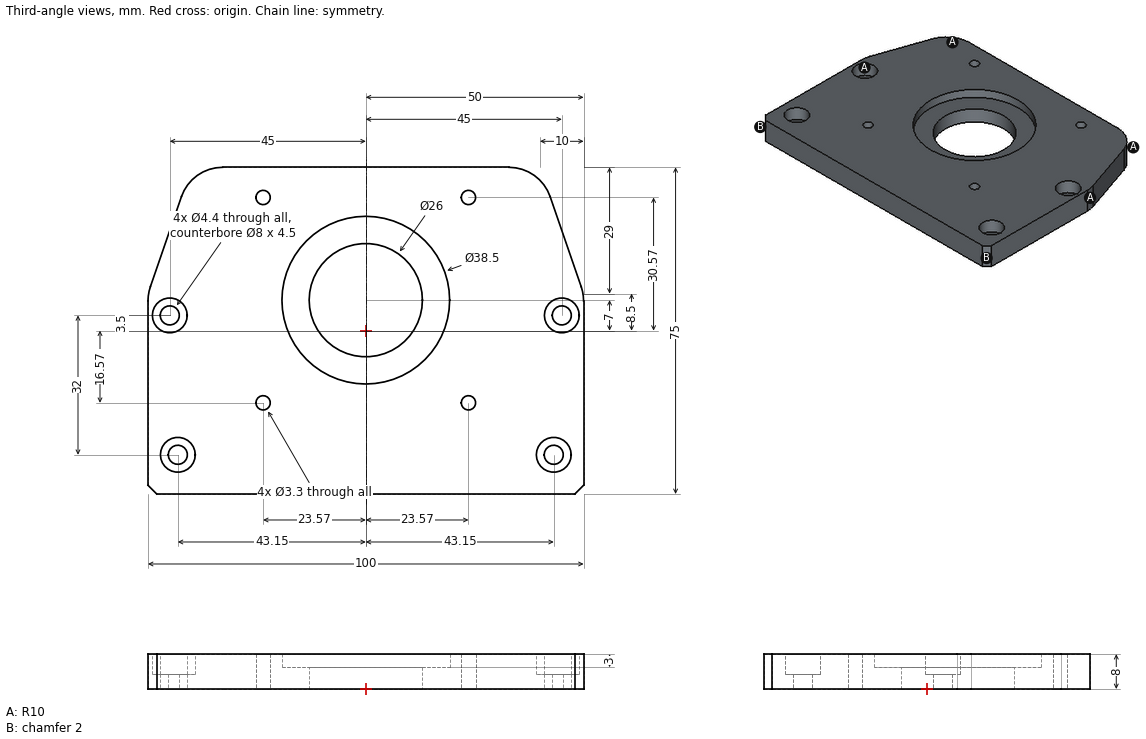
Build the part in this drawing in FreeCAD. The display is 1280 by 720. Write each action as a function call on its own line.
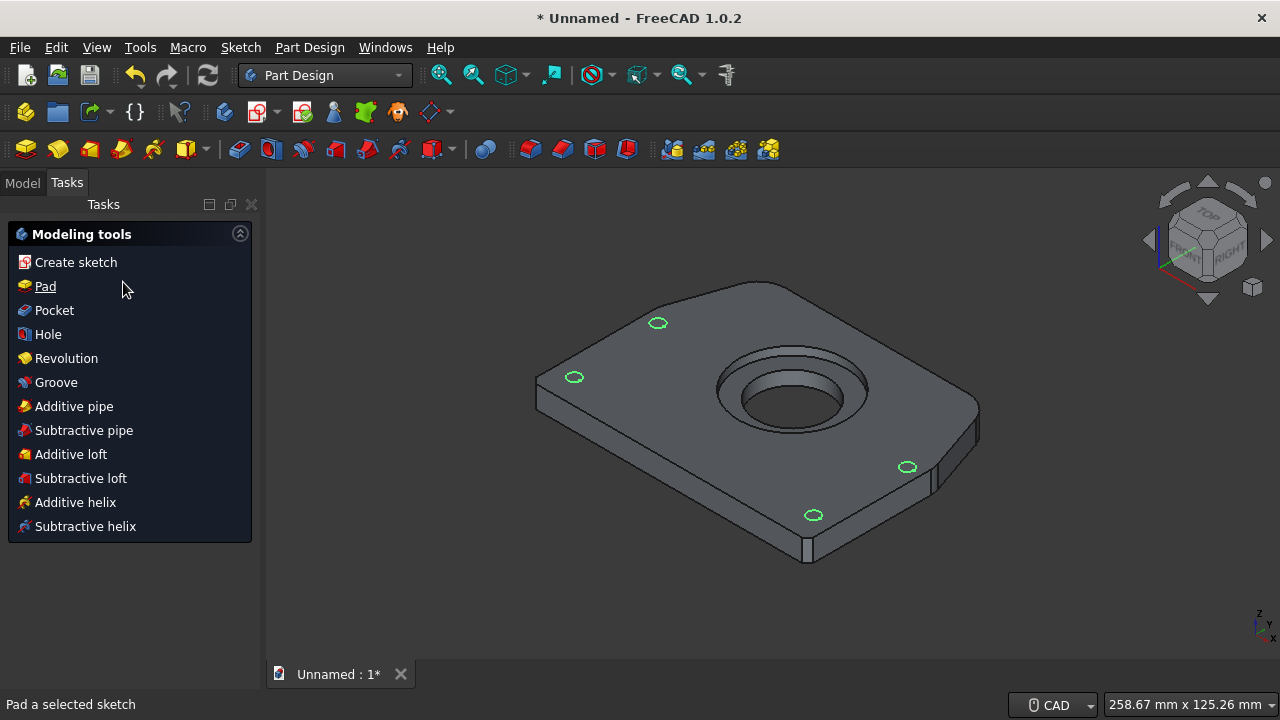
click(272, 150)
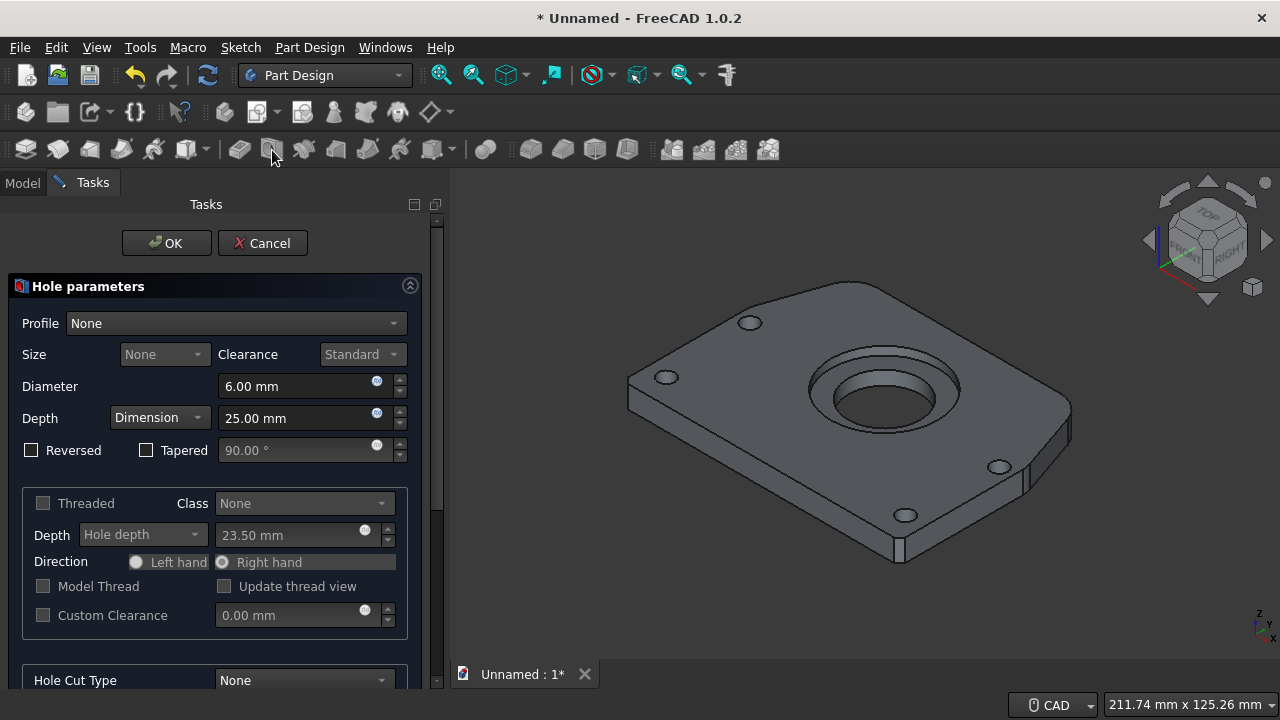
triple_click(305, 386)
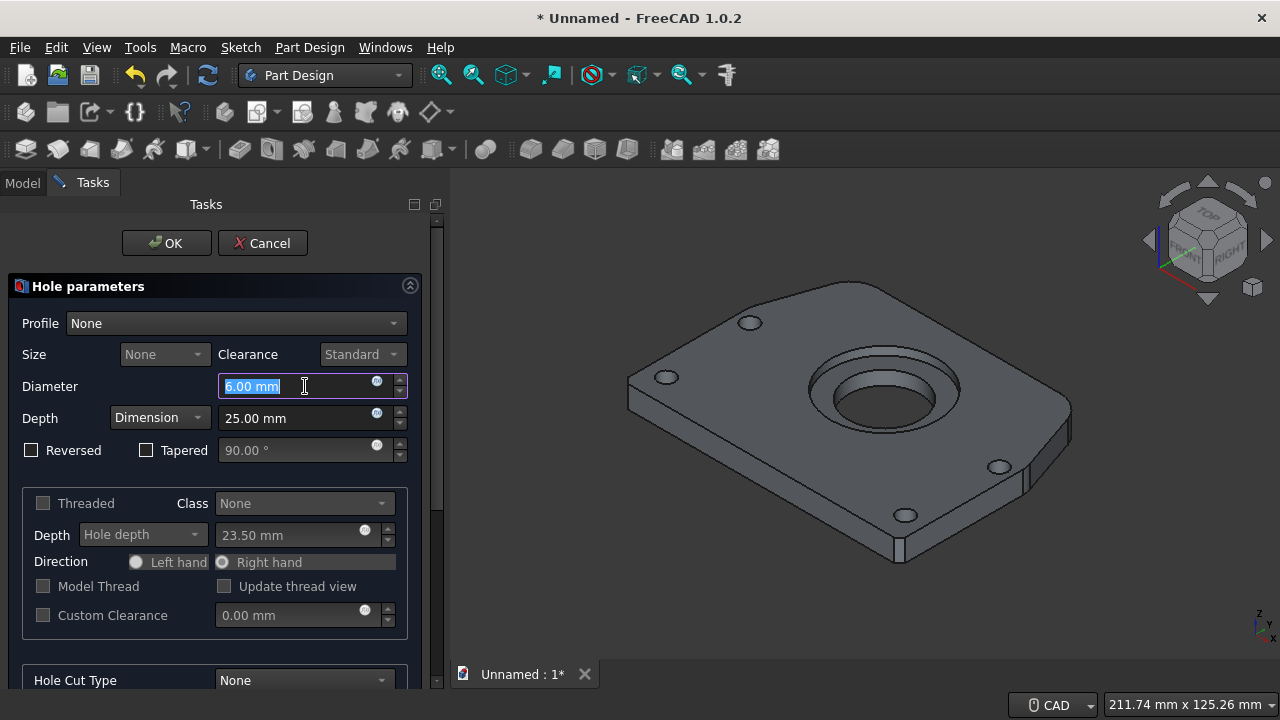
text(4.4)
key(Tab)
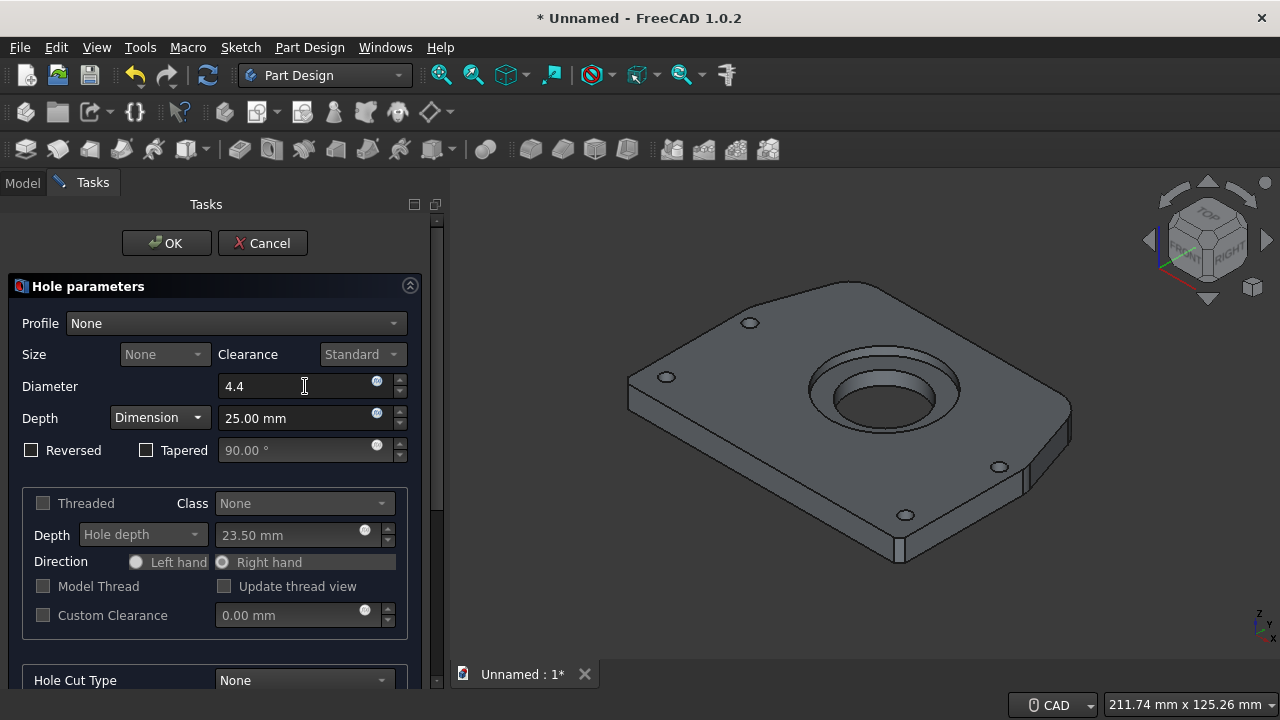
click(161, 418)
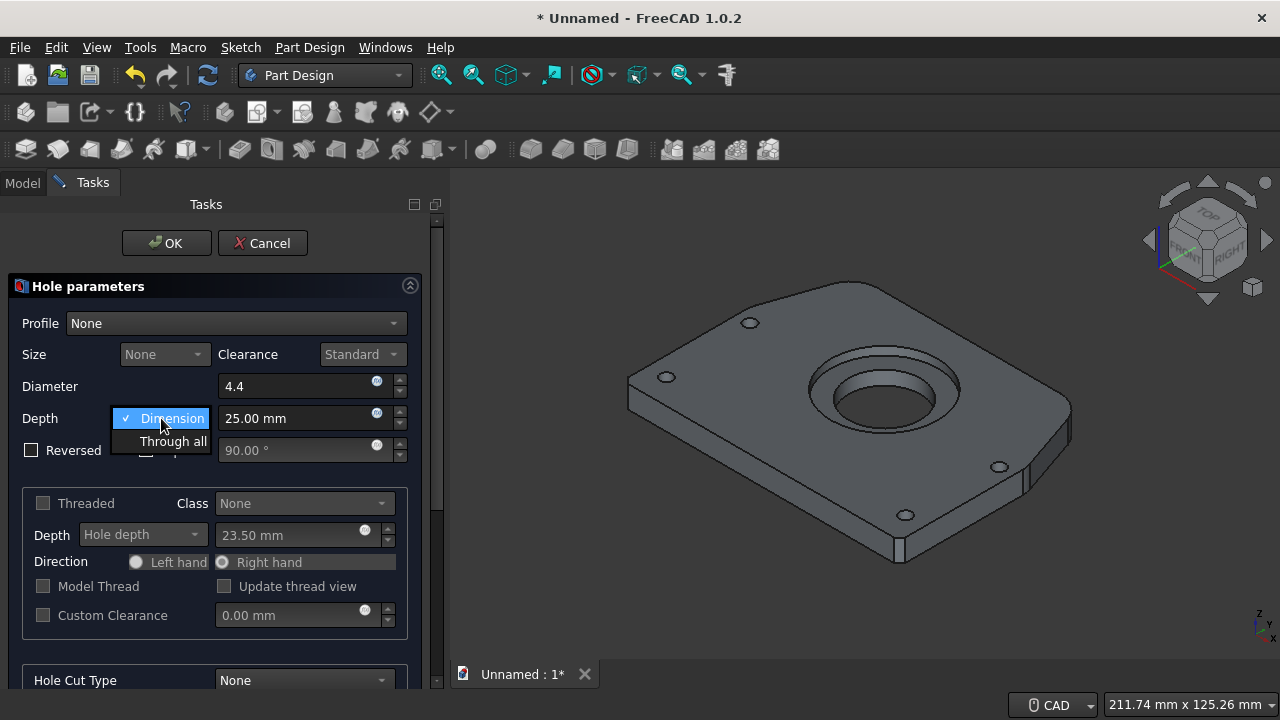
click(160, 442)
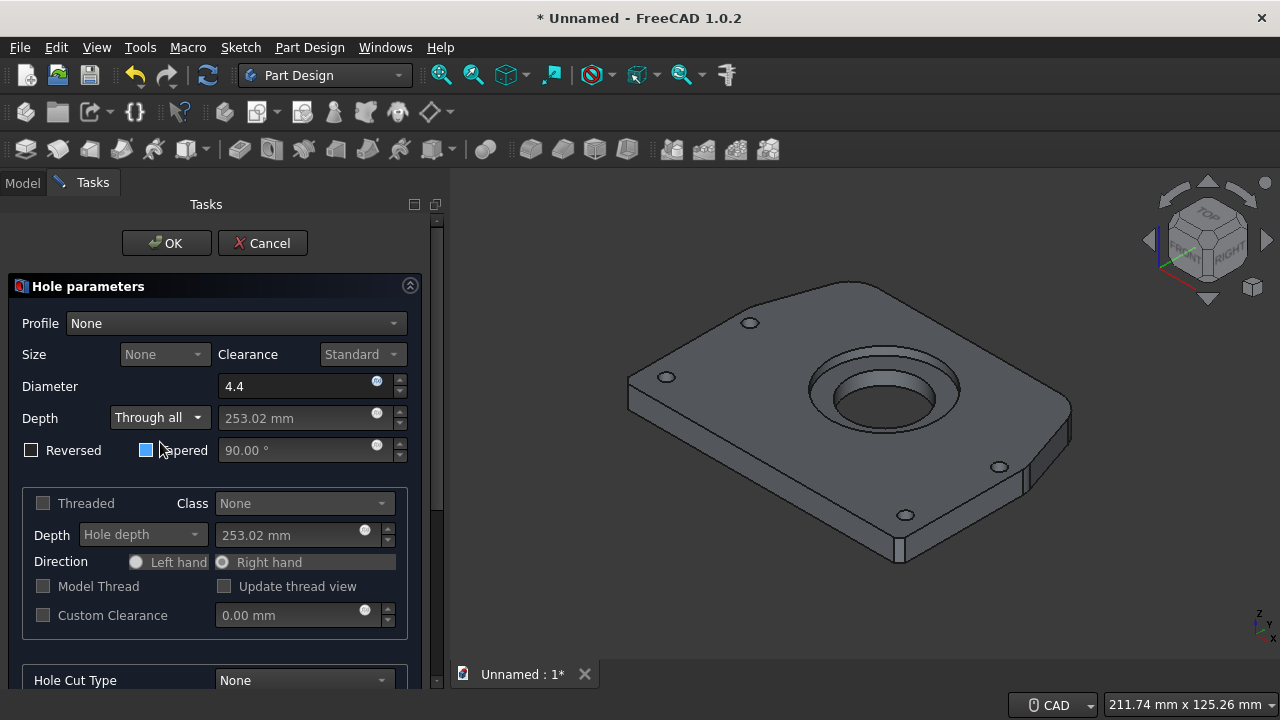
scroll(437, 451, down, 2)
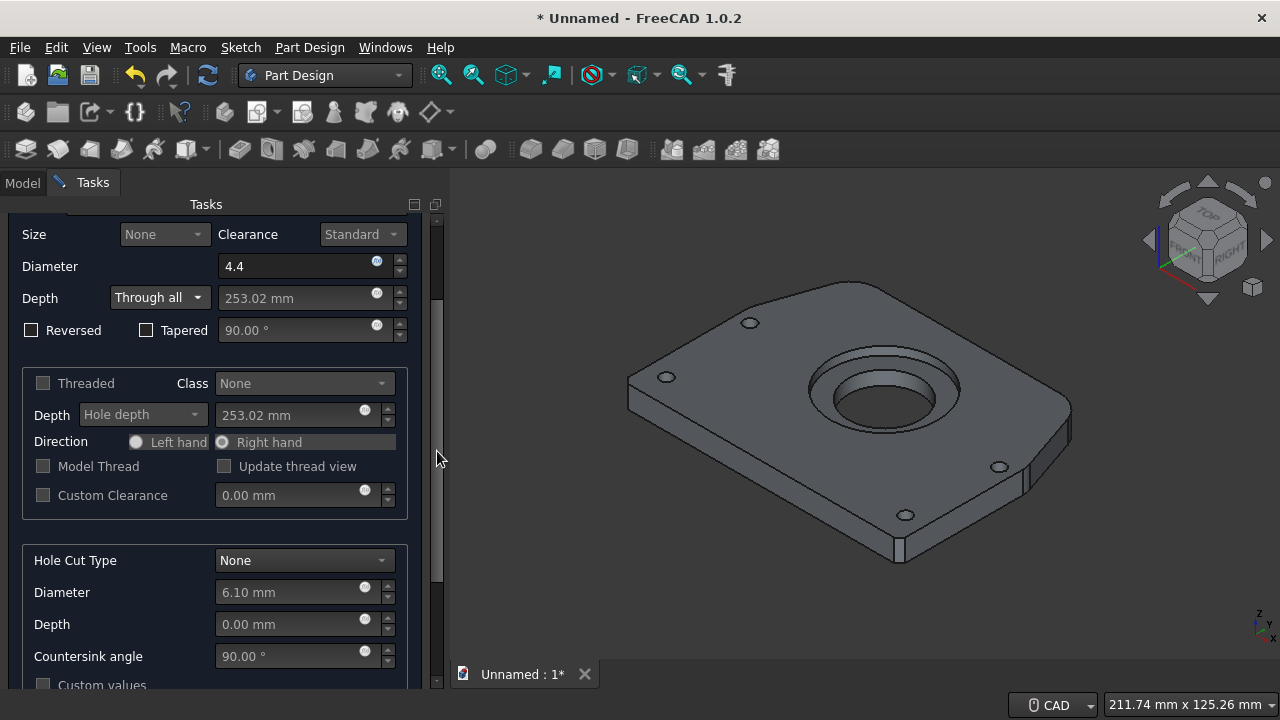
click(306, 560)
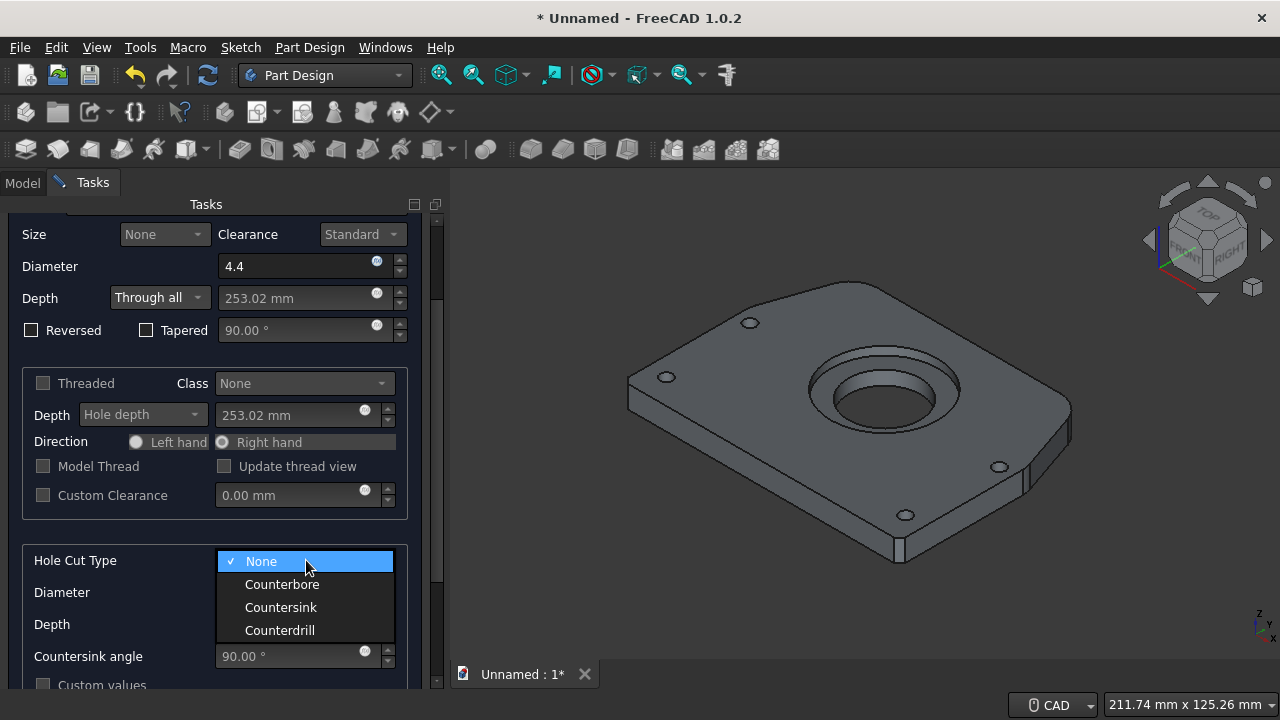
click(304, 584)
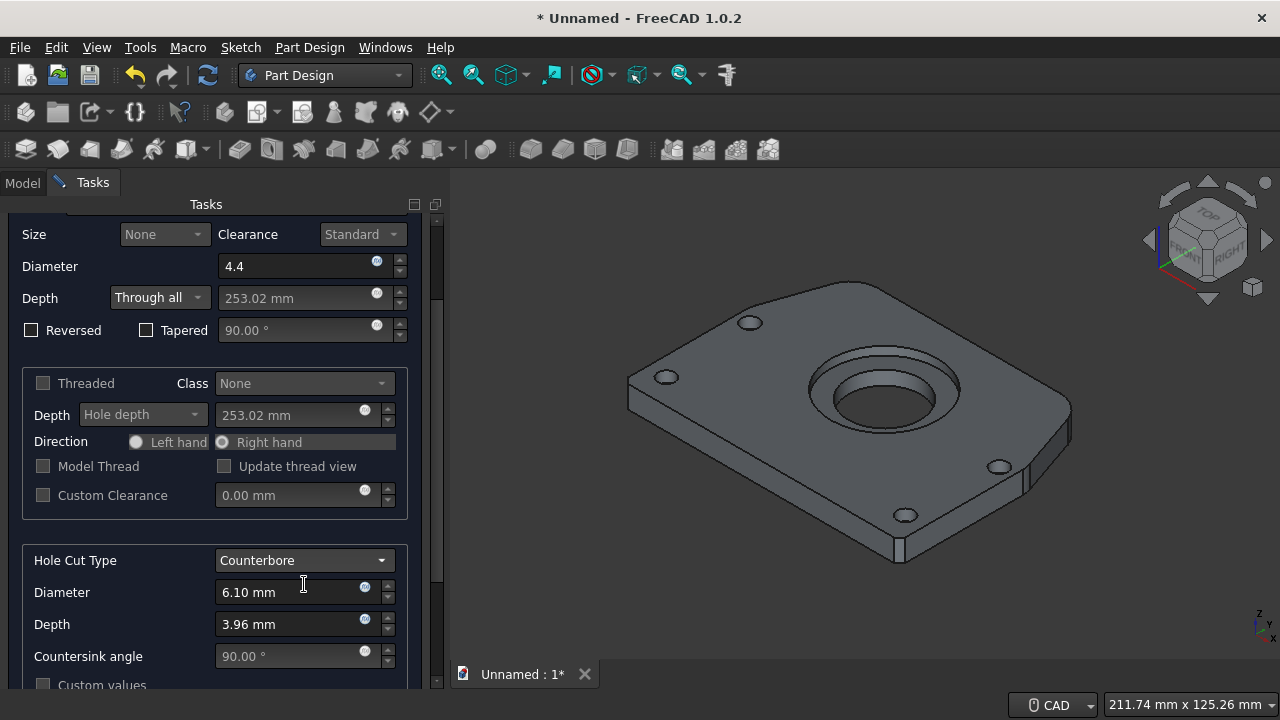
triple_click(298, 592)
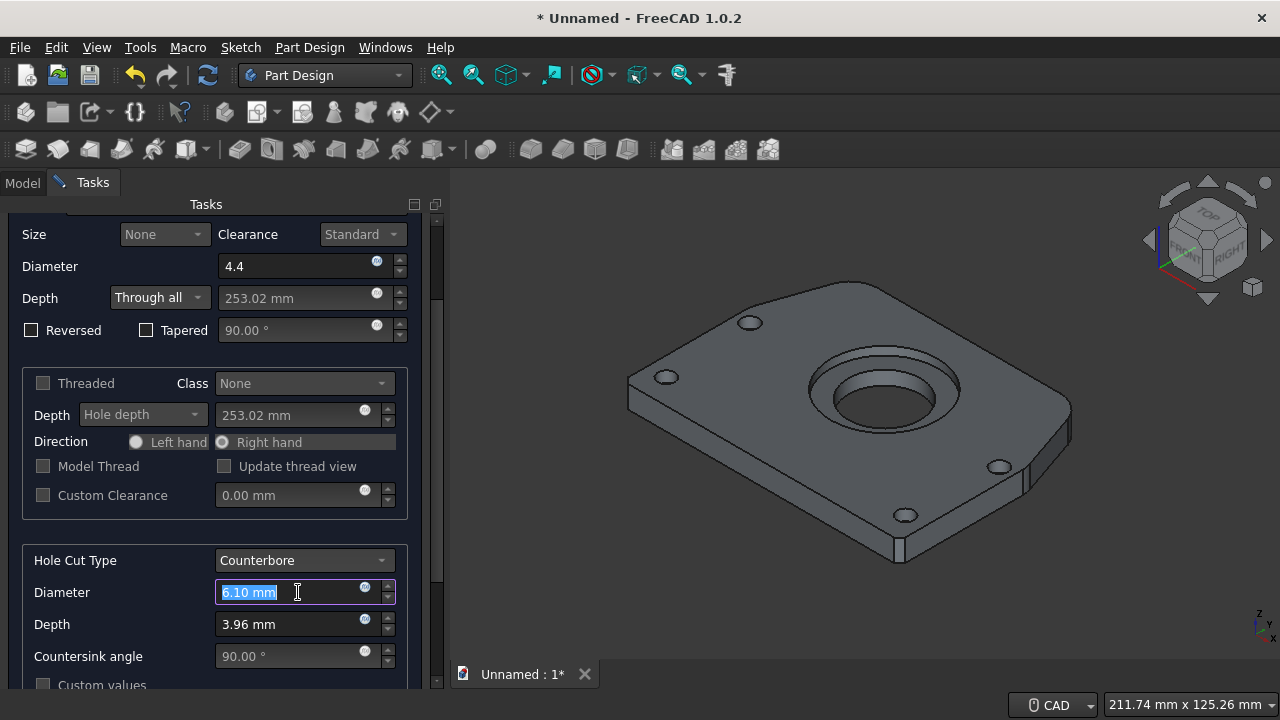
text(8)
key(Tab)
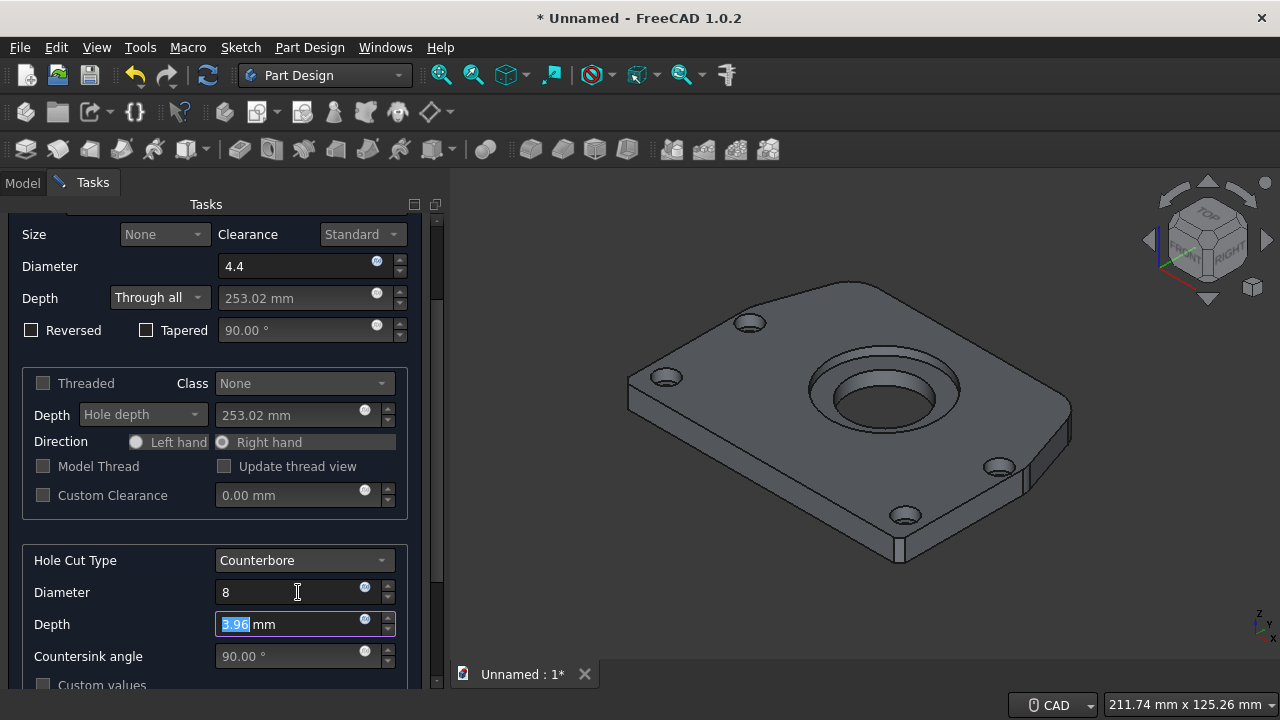
text(4.5)
key(Tab)